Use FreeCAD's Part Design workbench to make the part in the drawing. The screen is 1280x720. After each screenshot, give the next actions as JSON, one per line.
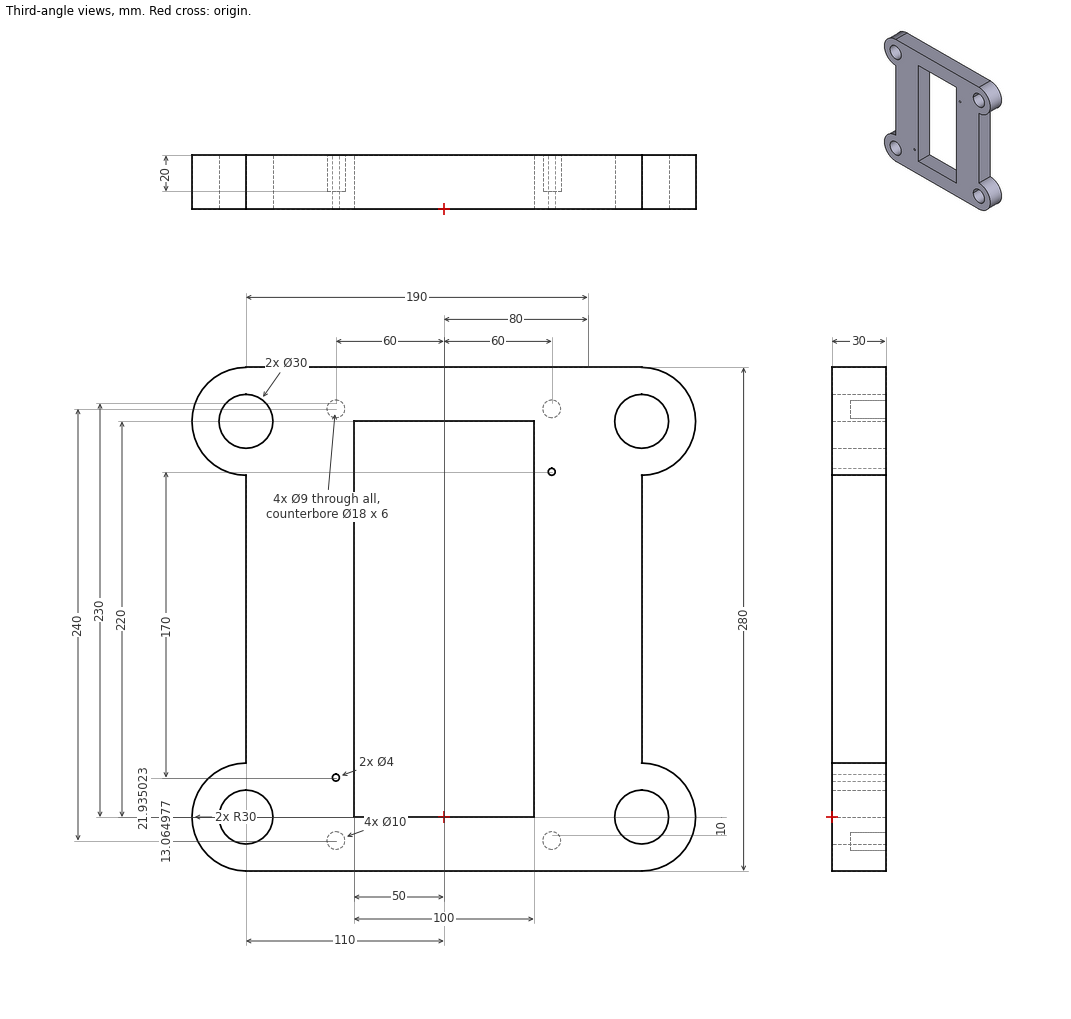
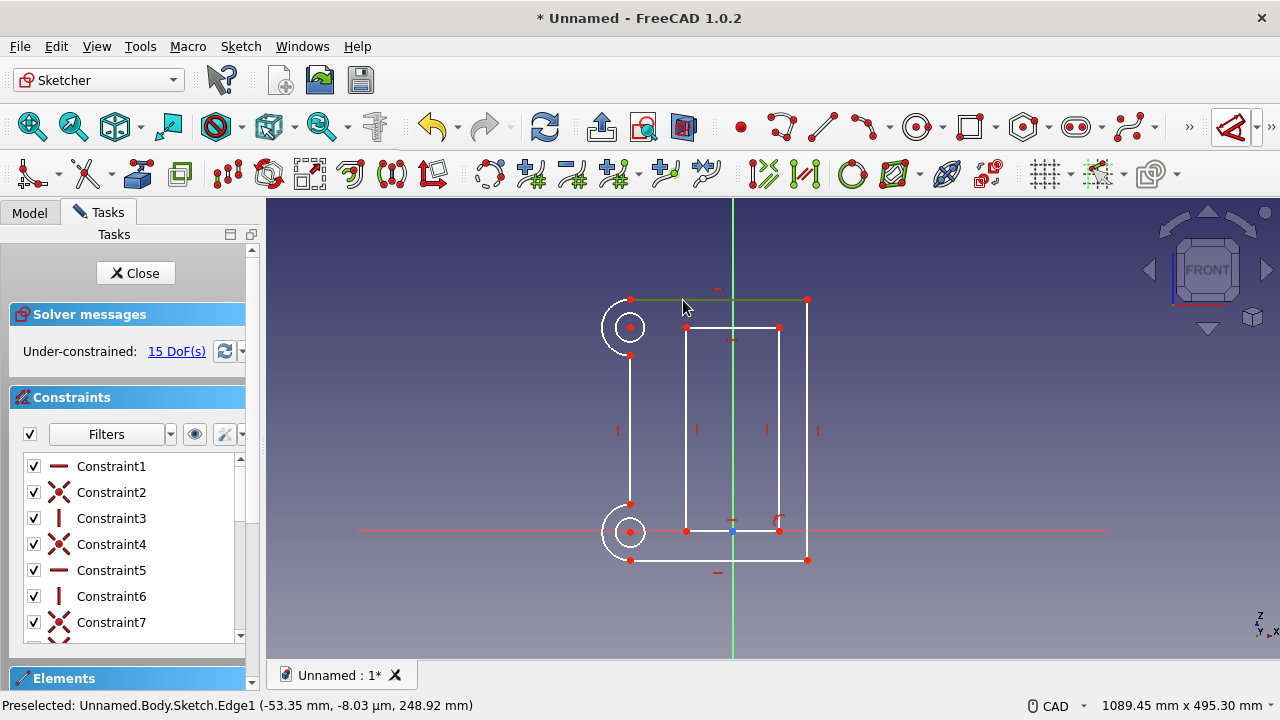
{"action": "left_click", "coordinate": [607, 311]}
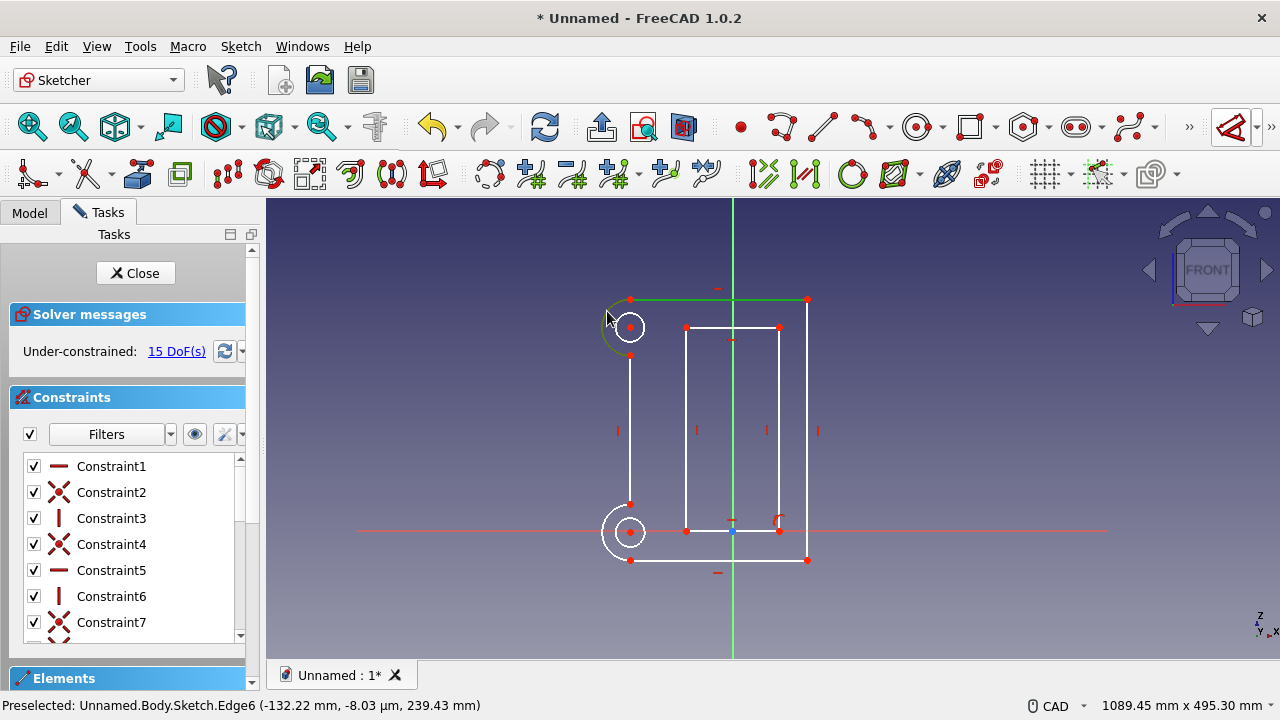
{"action": "key", "text": "t"}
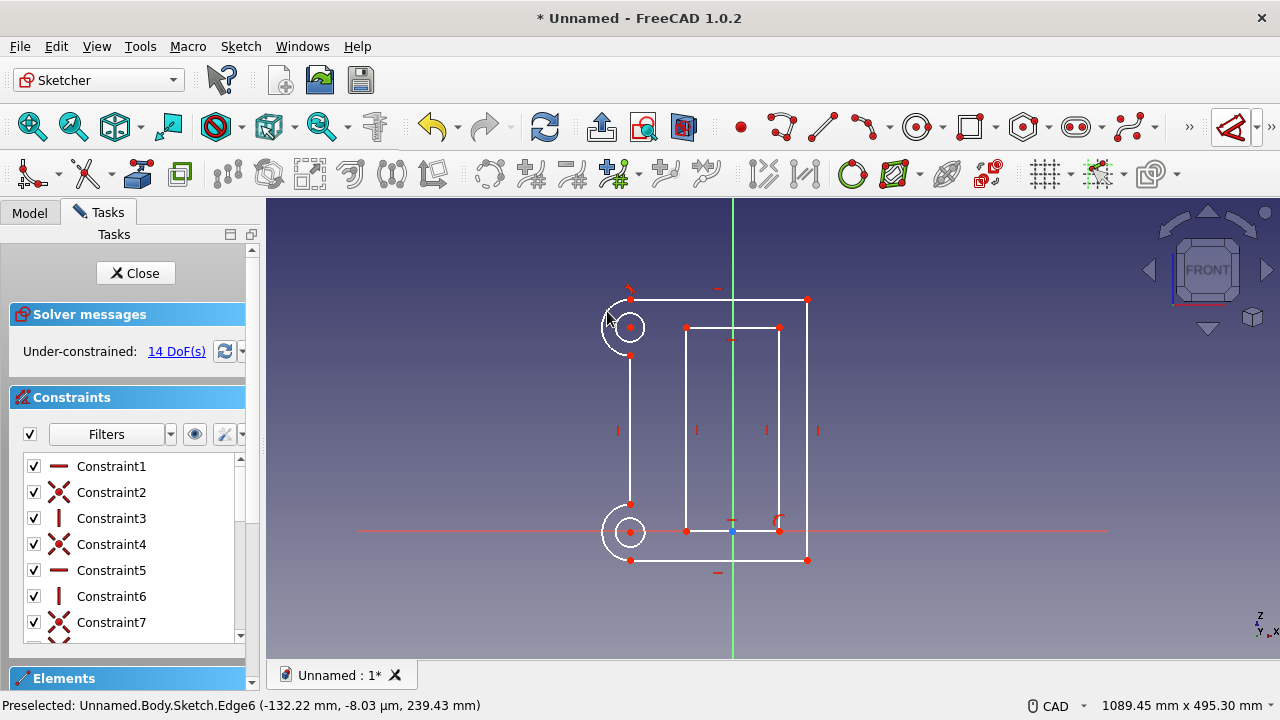
{"action": "left_click", "coordinate": [754, 561]}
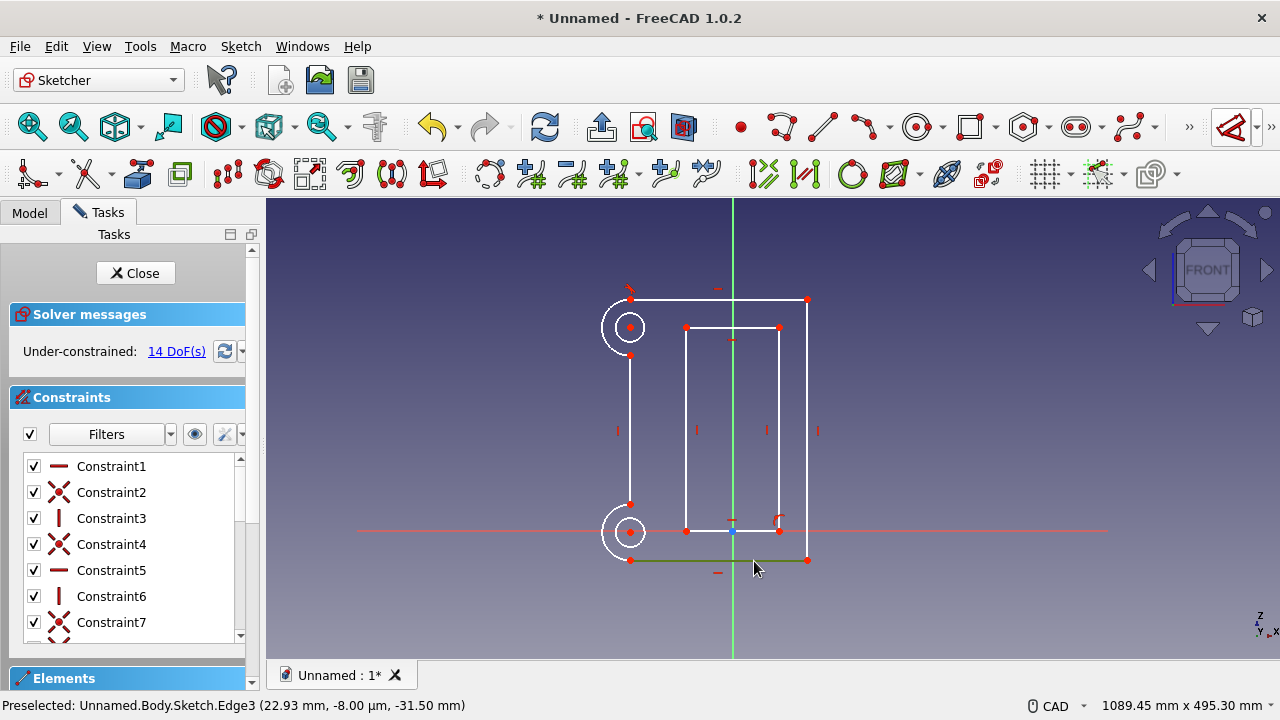
{"action": "left_click", "coordinate": [608, 516]}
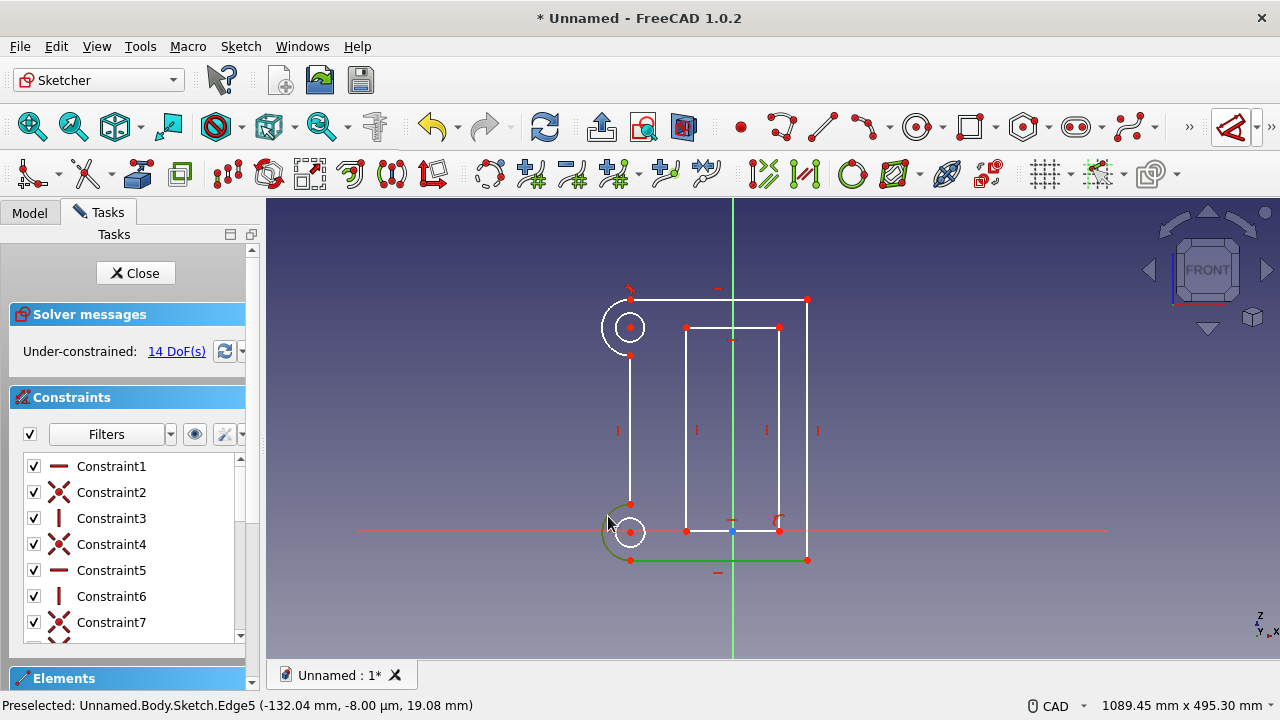
{"action": "key", "text": "t"}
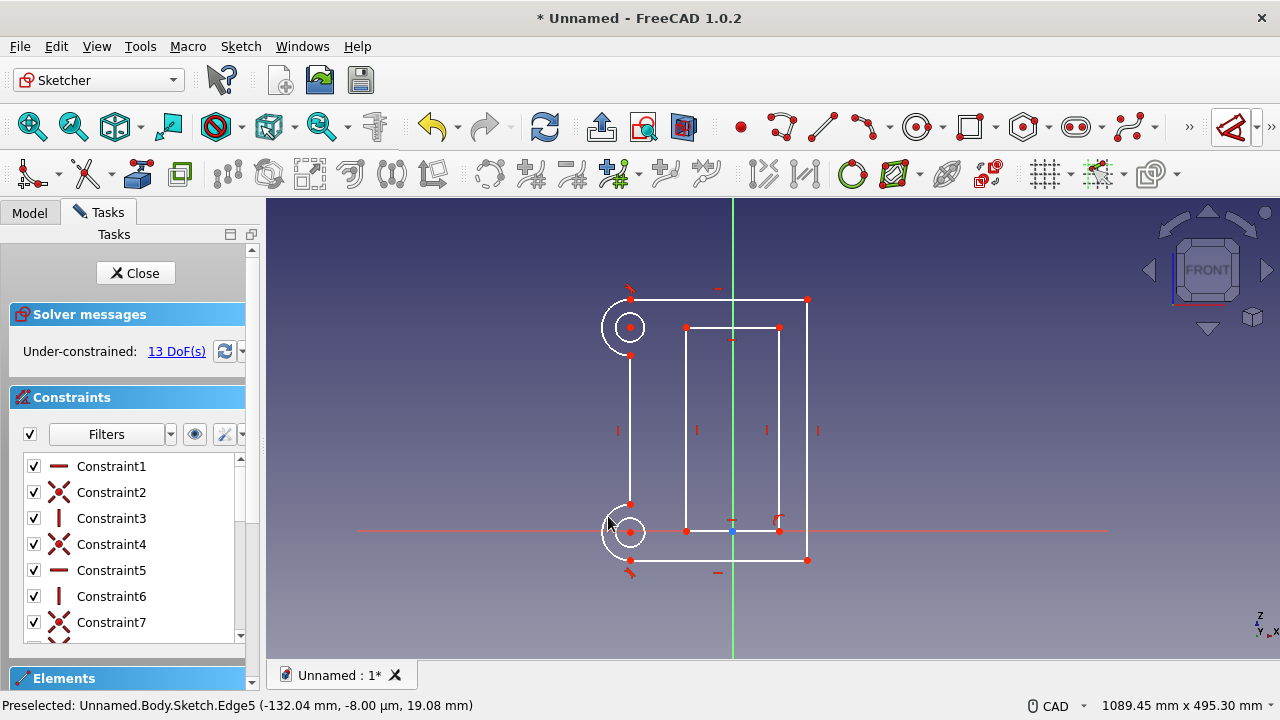
{"action": "left_click", "coordinate": [607, 516]}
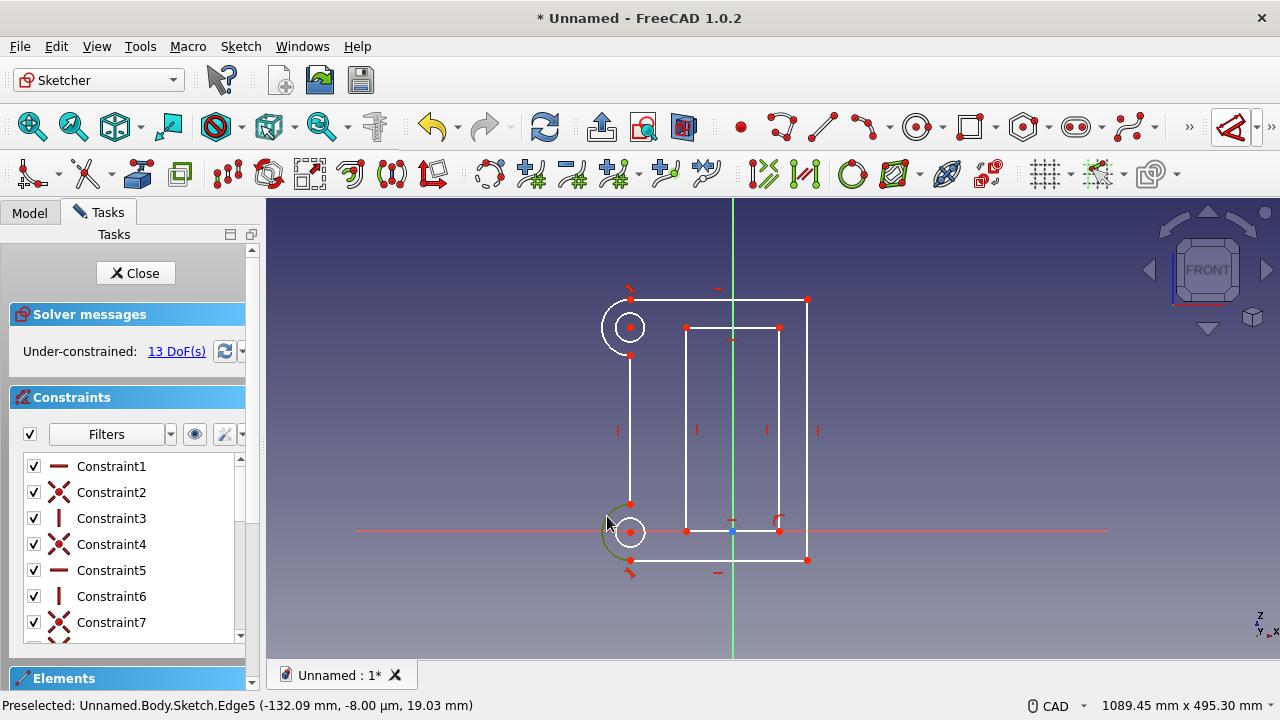
{"action": "left_click", "coordinate": [607, 311]}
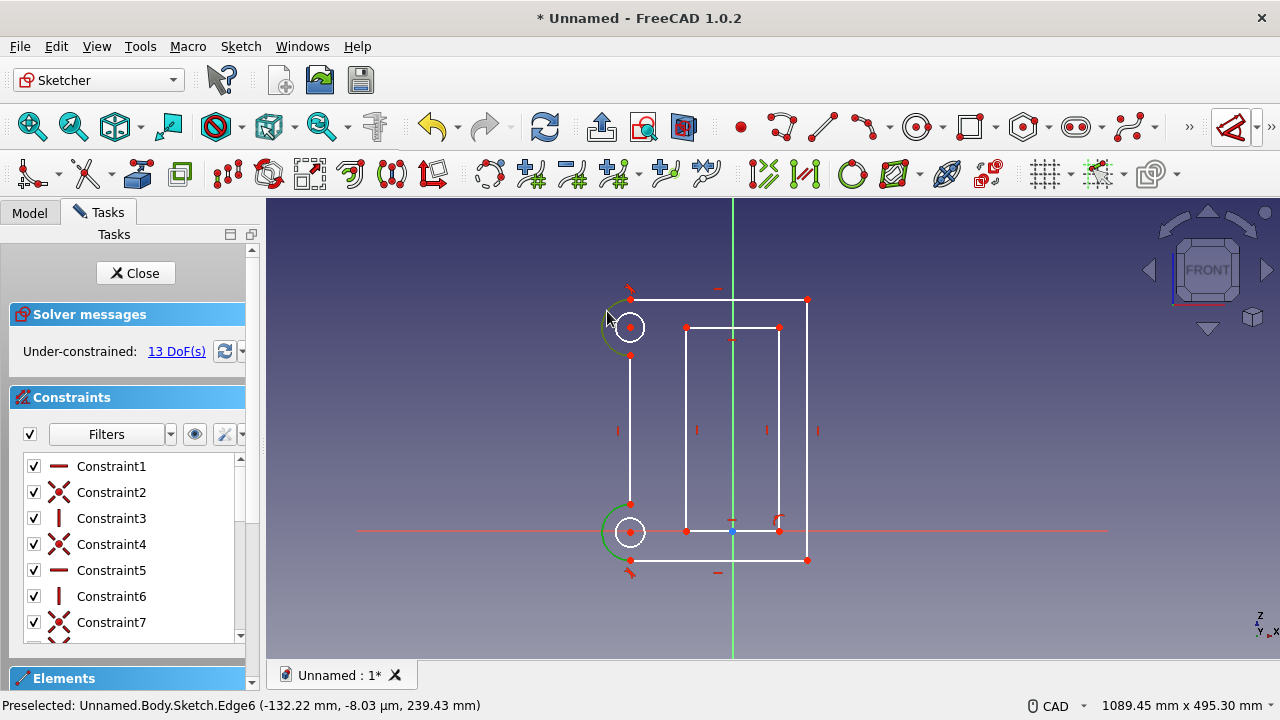
{"action": "key", "text": "e"}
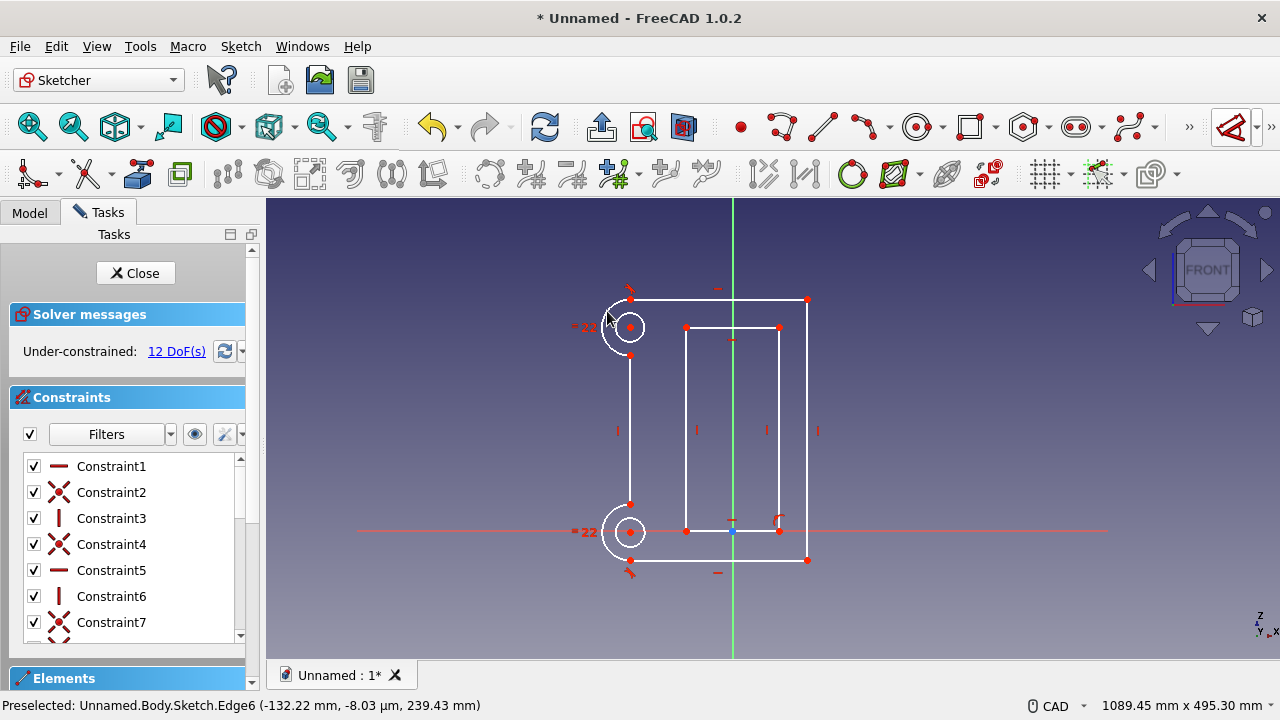
{"action": "left_click", "coordinate": [640, 317]}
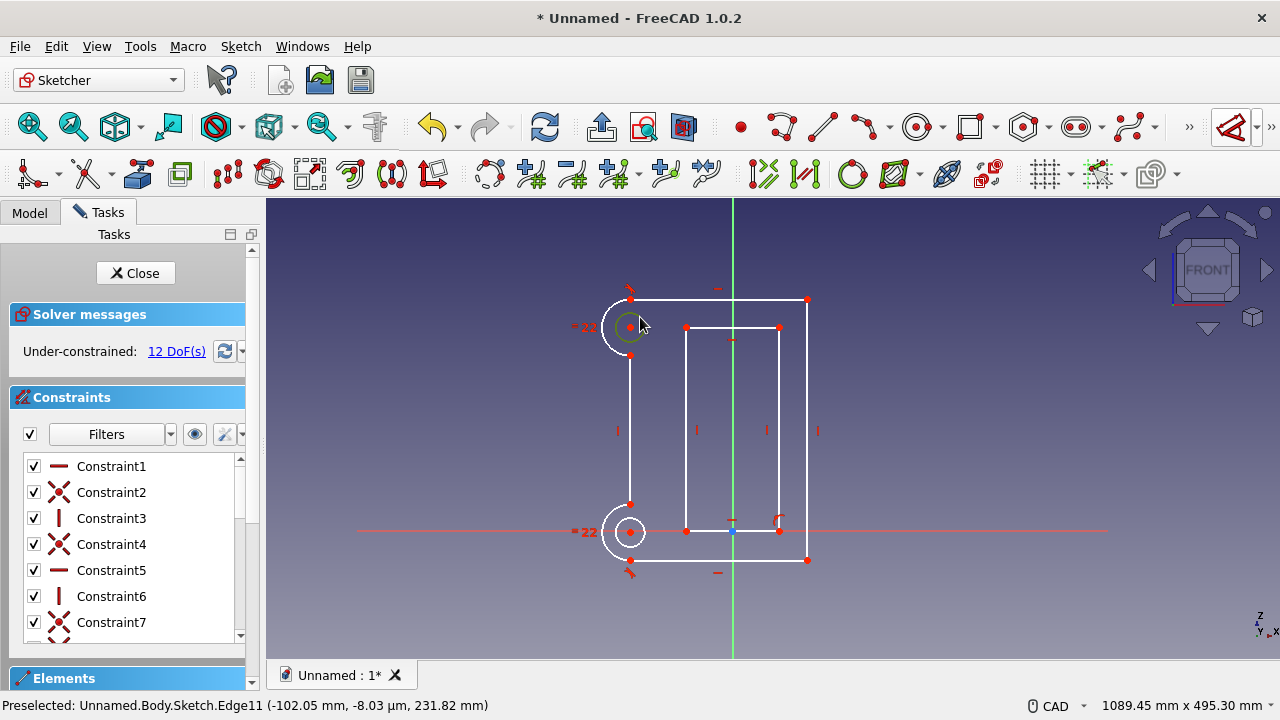
{"action": "left_click", "coordinate": [620, 543]}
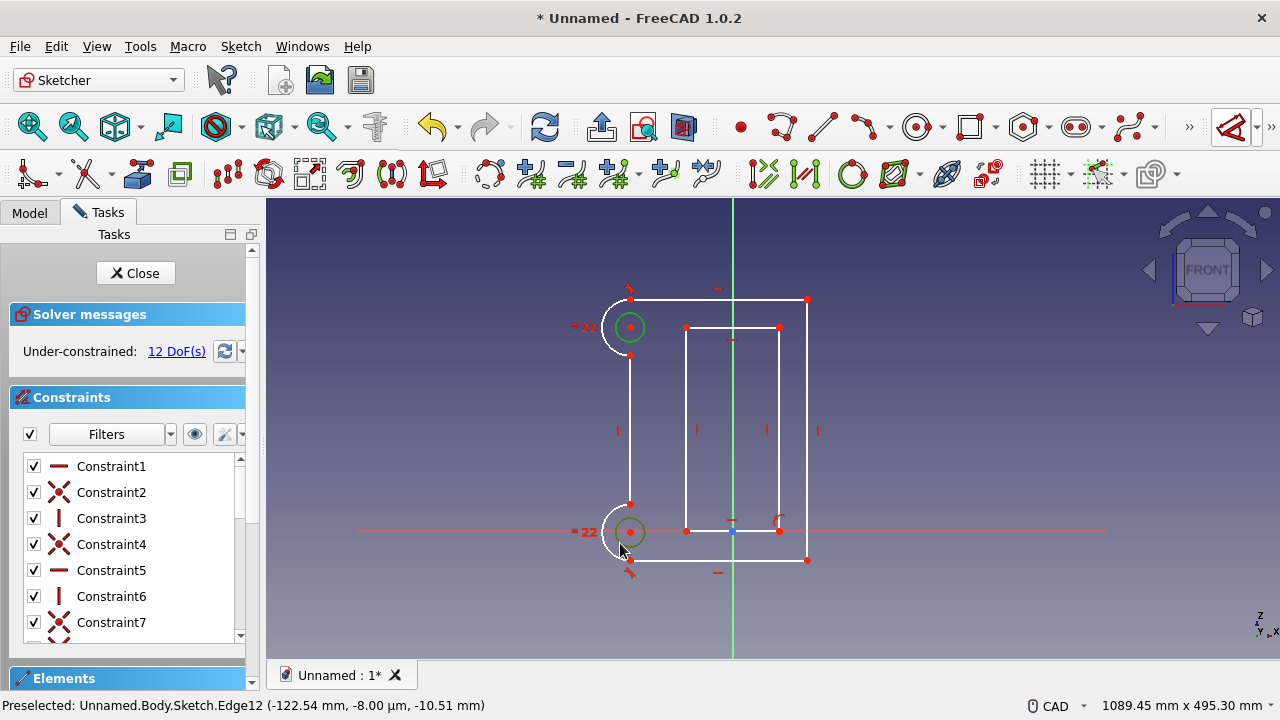
{"action": "key", "text": "e"}